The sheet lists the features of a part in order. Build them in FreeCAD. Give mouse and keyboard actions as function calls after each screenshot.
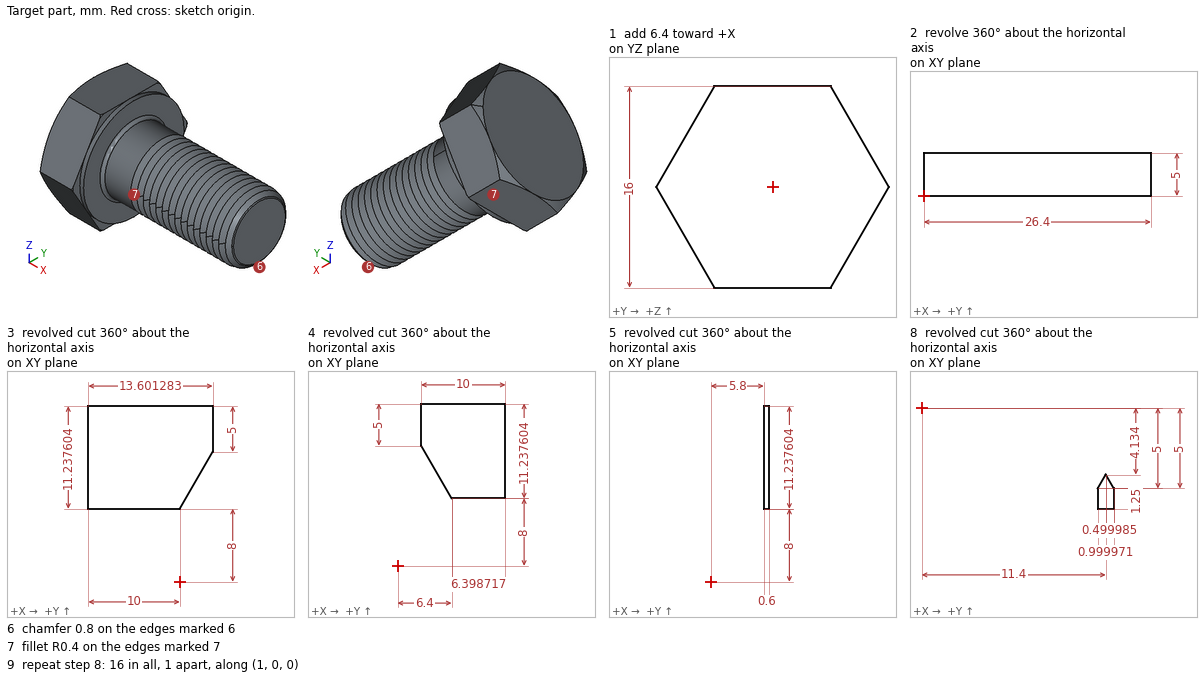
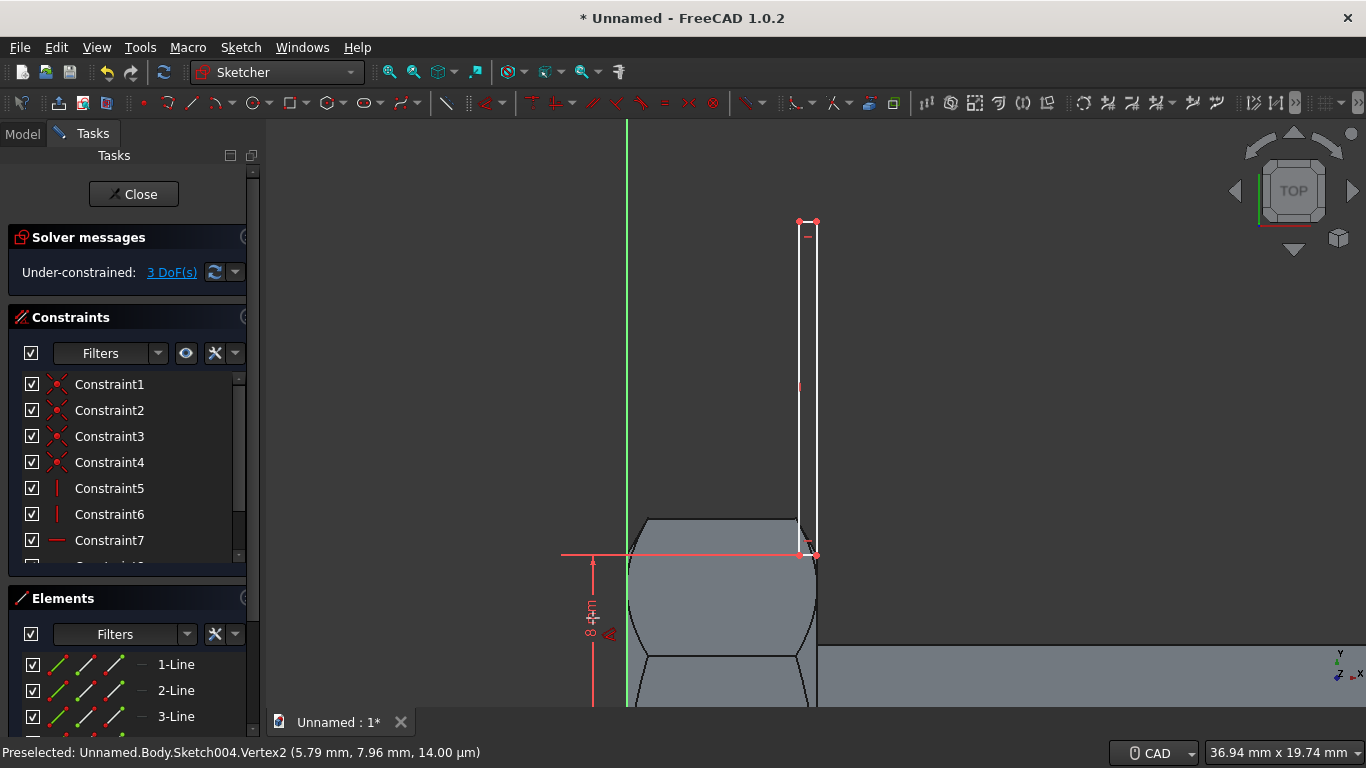
scroll(808, 555, up, 4)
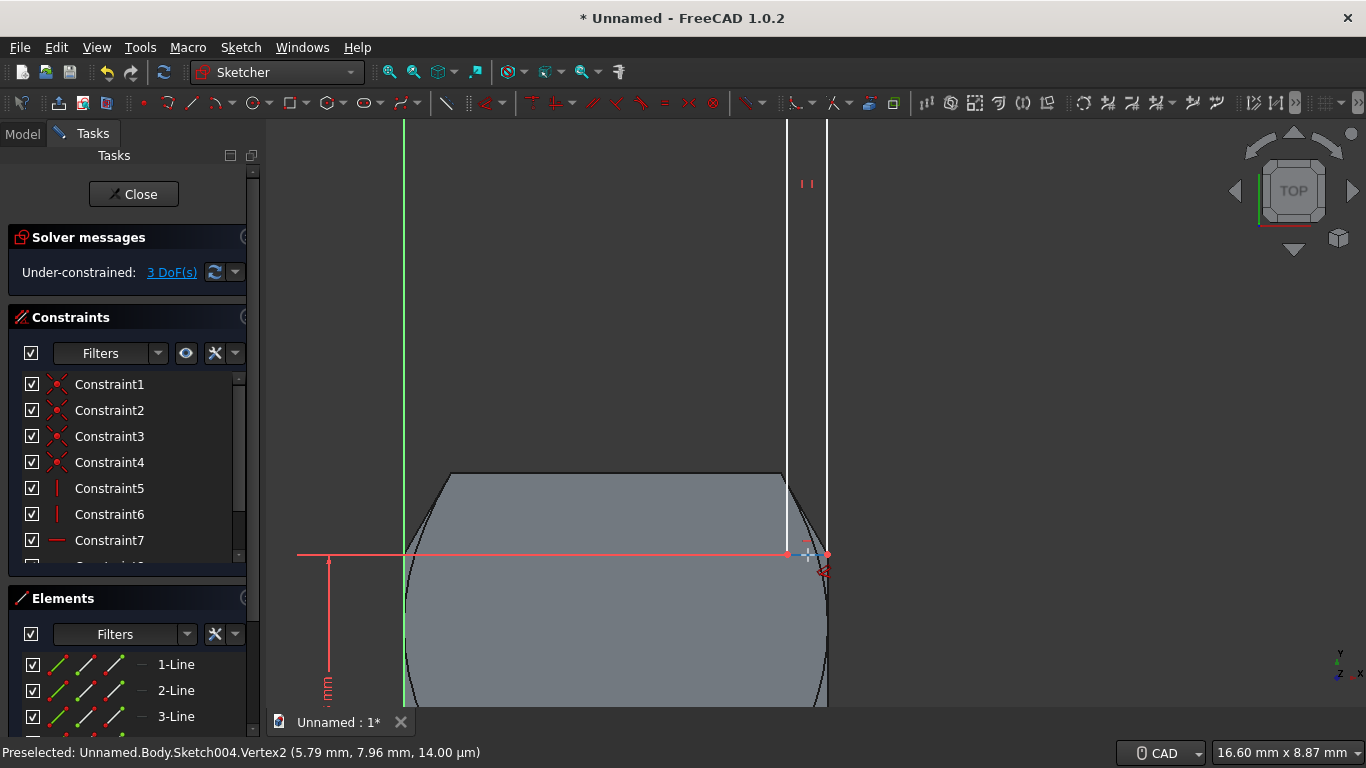
click(807, 555)
click(807, 589)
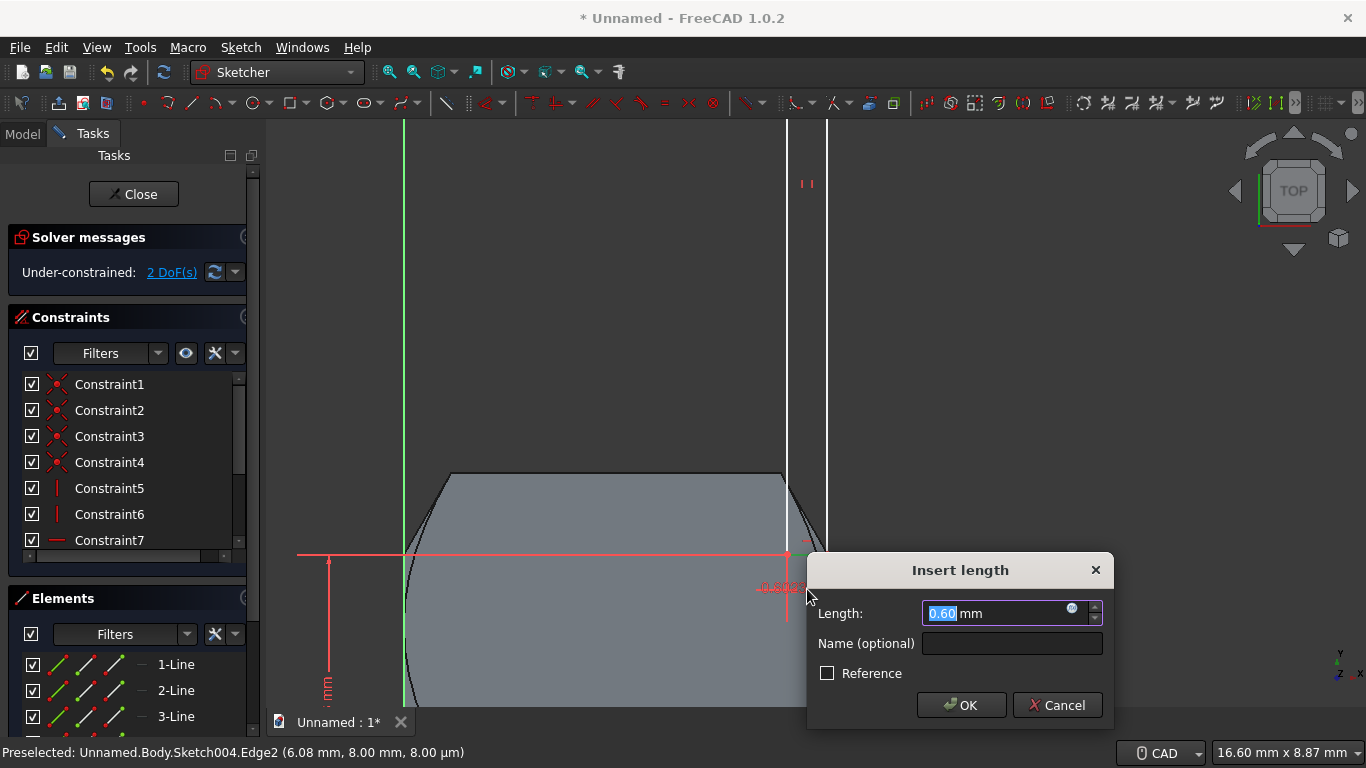
text(0.6)
key(Return)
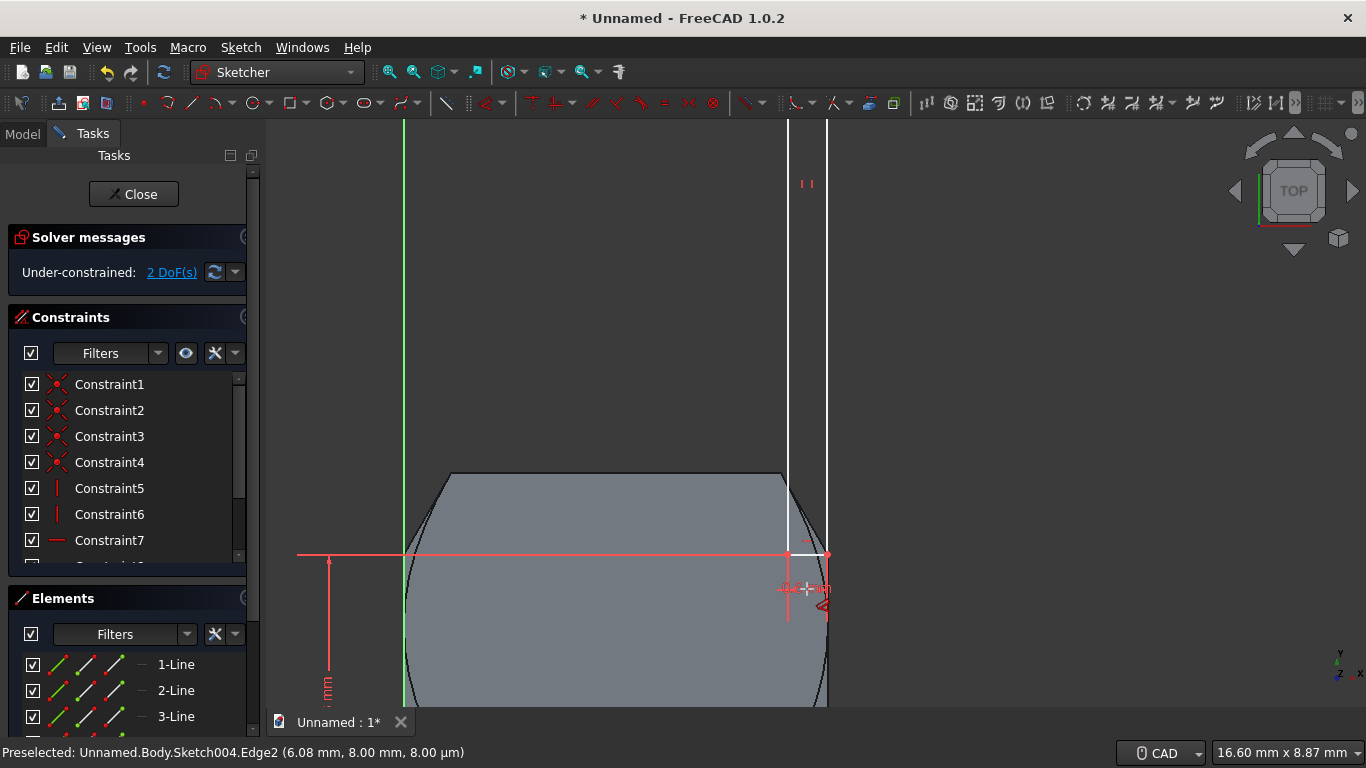
scroll(804, 398, down, 6)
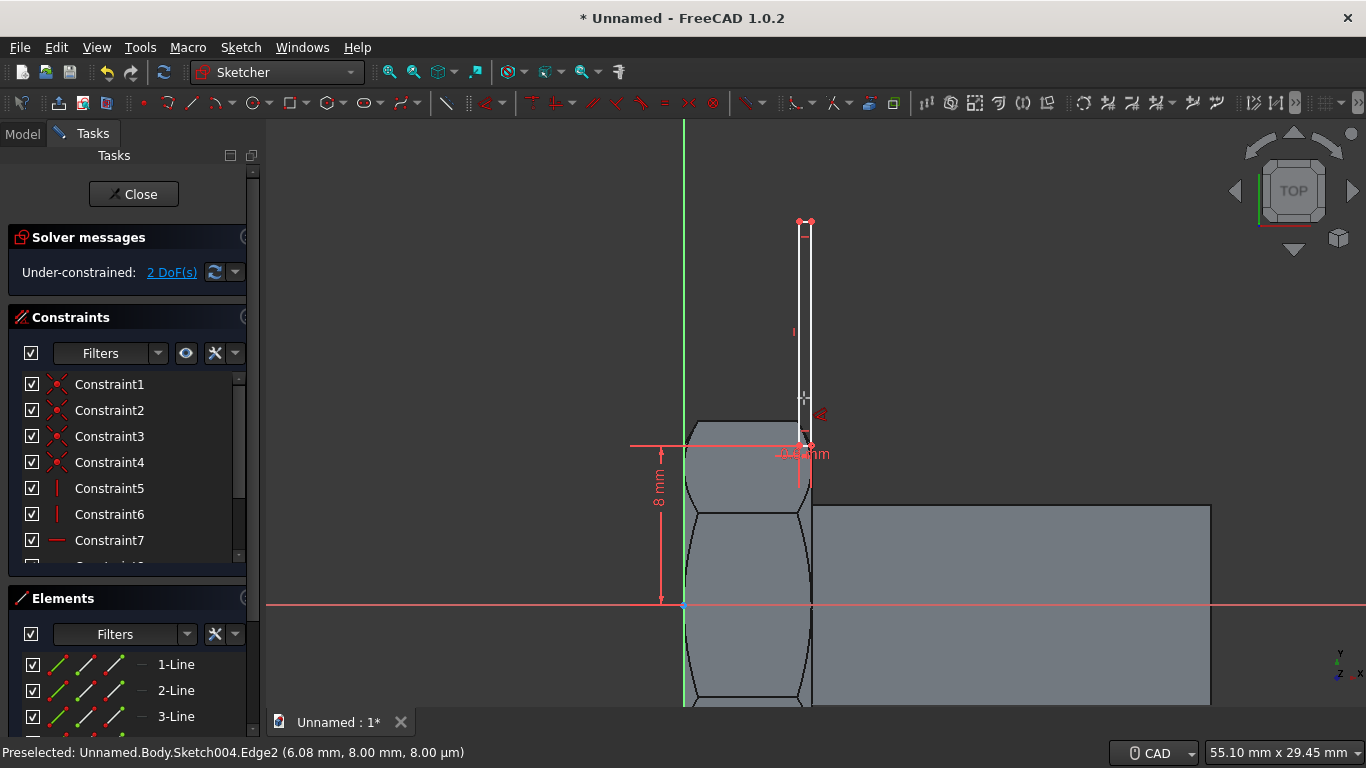
click(799, 222)
click(742, 639)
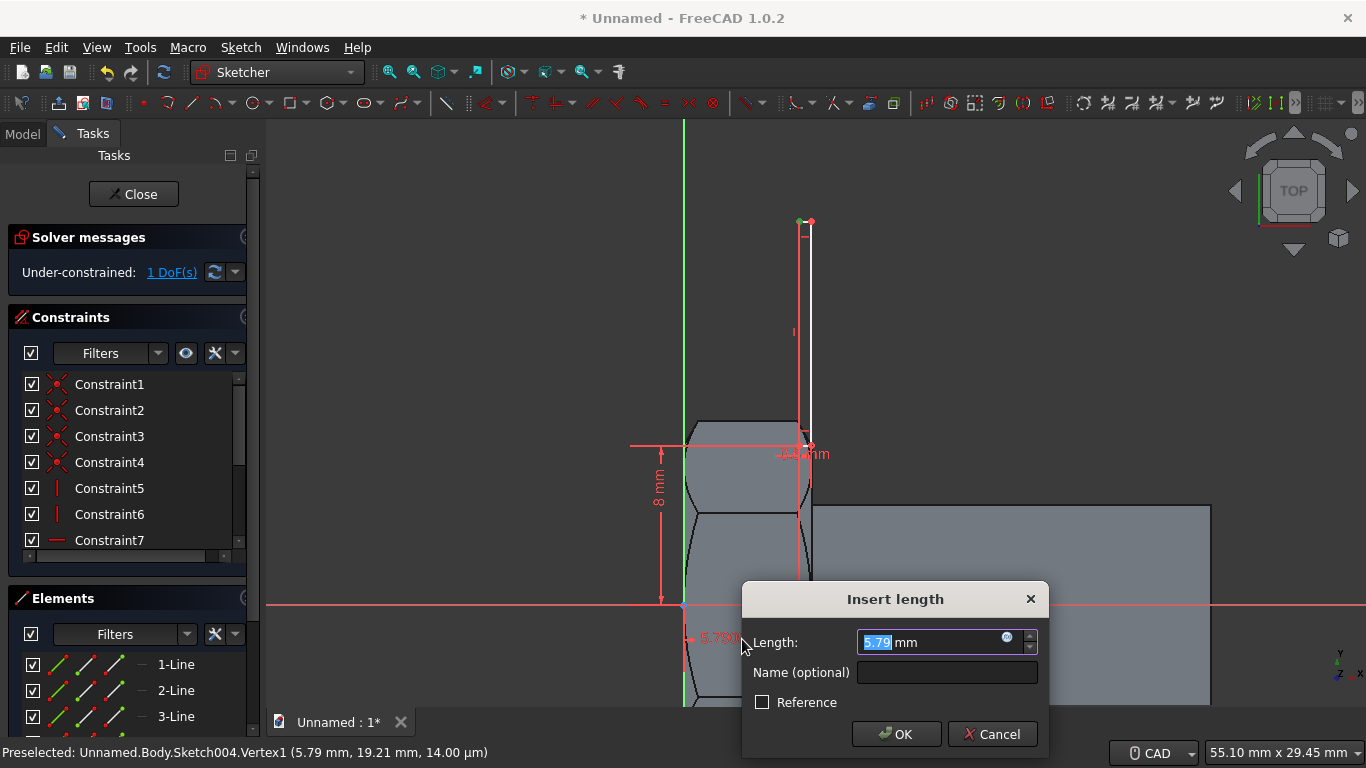
text(5.8)
key(Return)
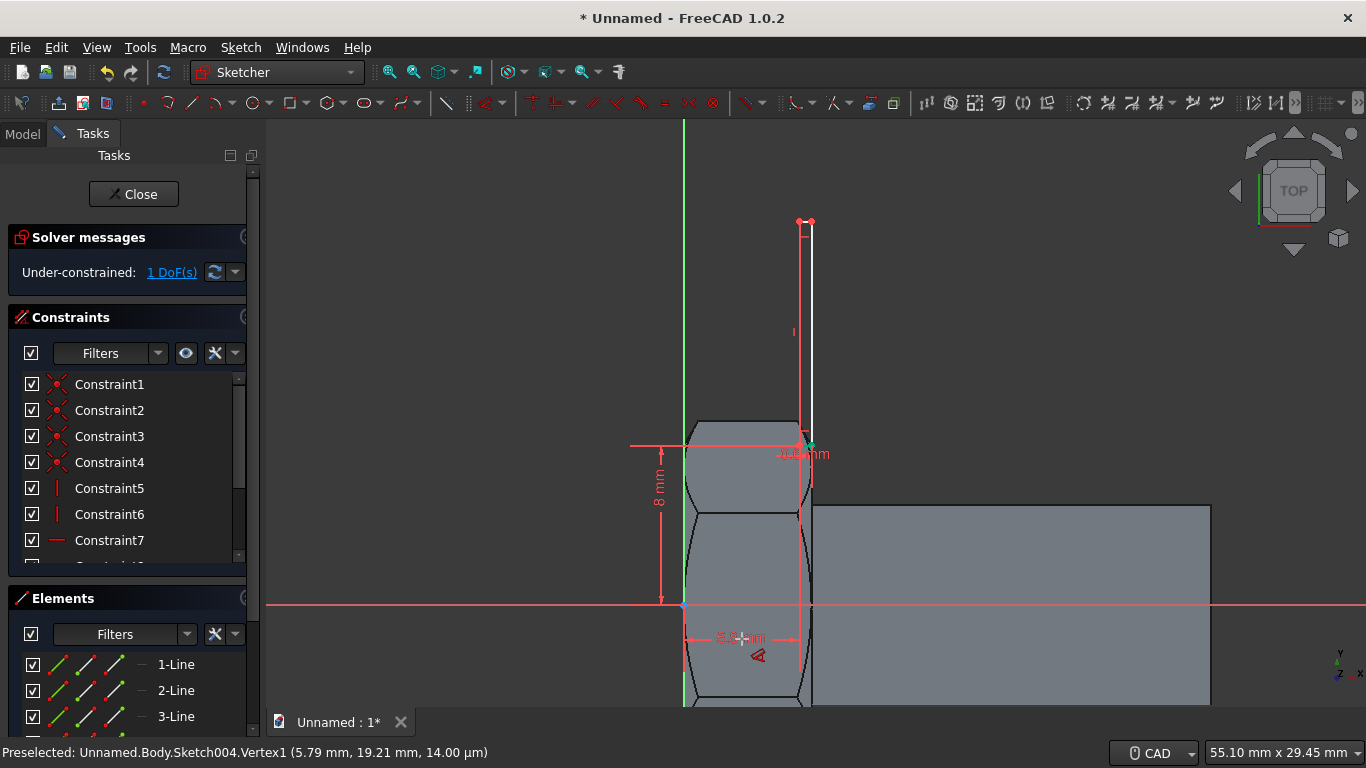
click(800, 289)
click(834, 334)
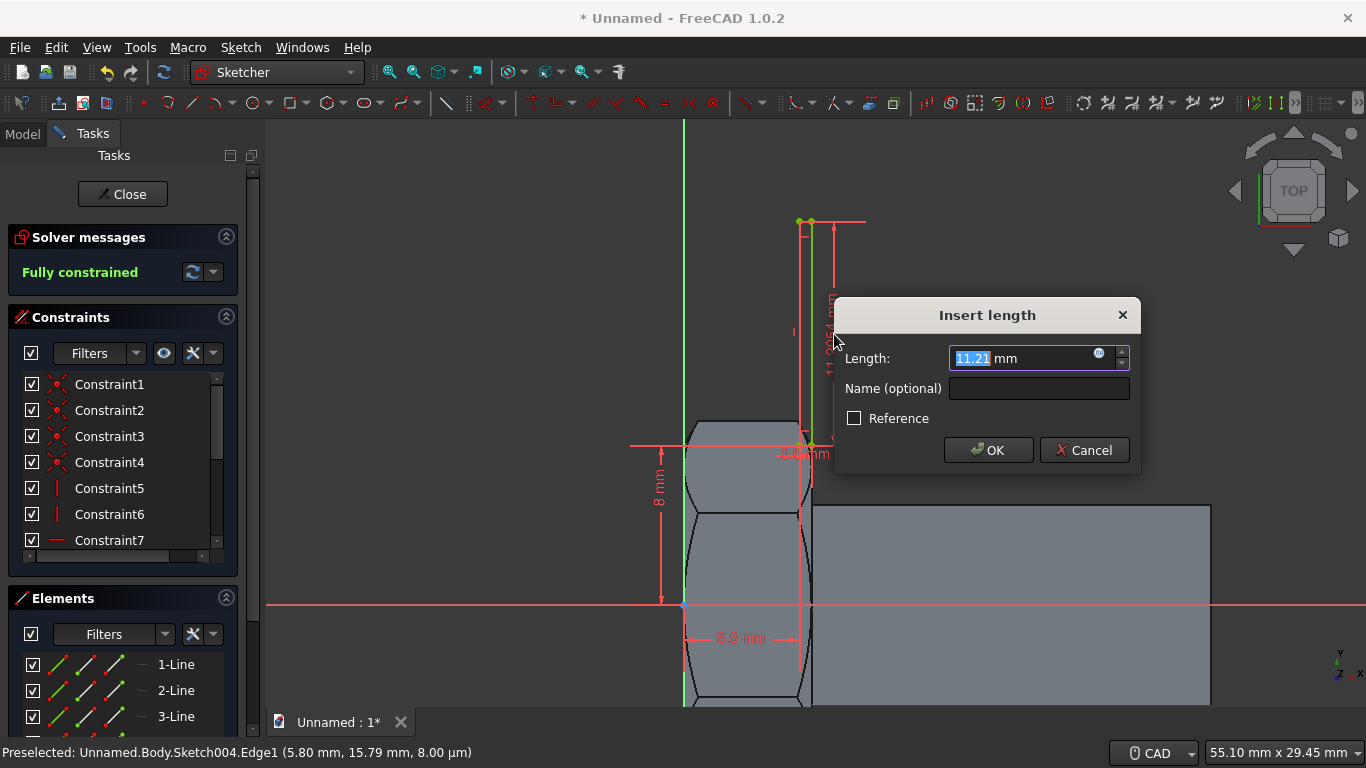
text(11.237604)
key(Return)
key(Escape)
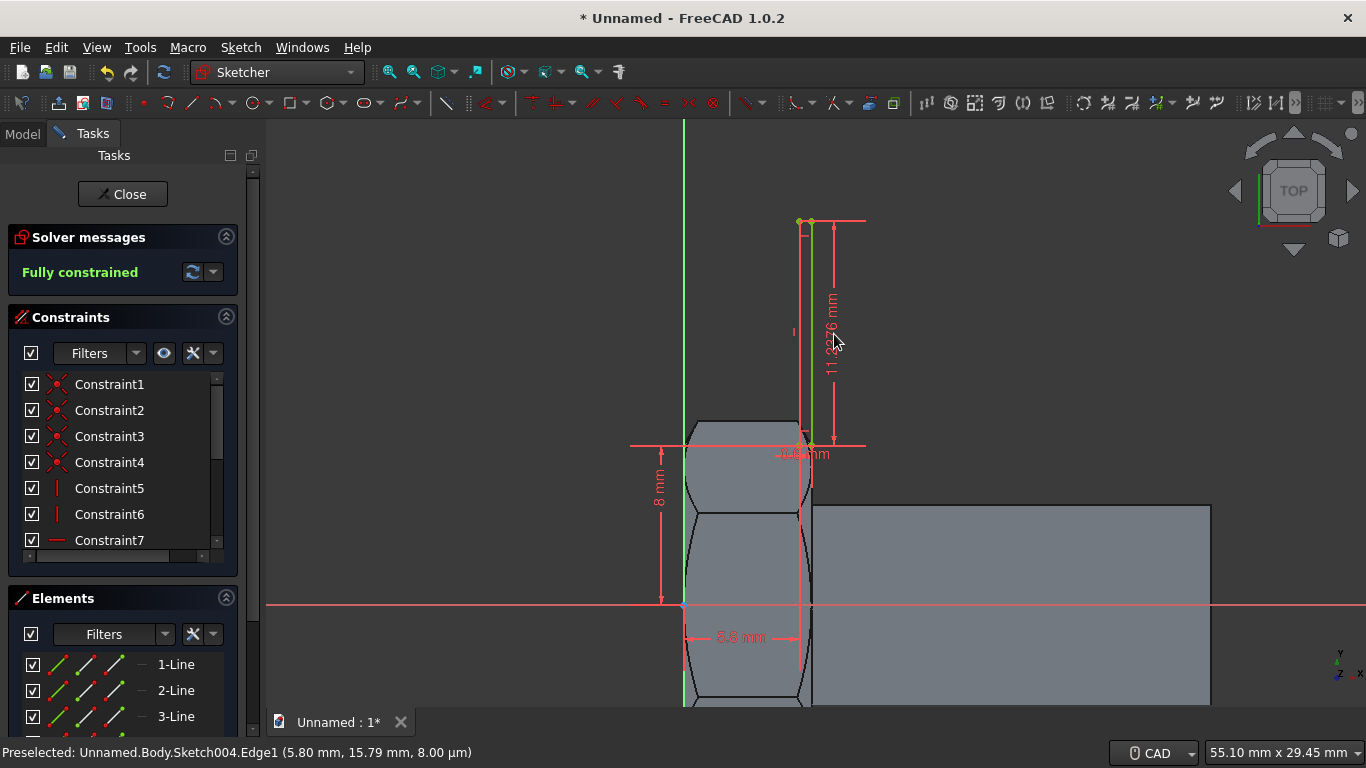
click(123, 194)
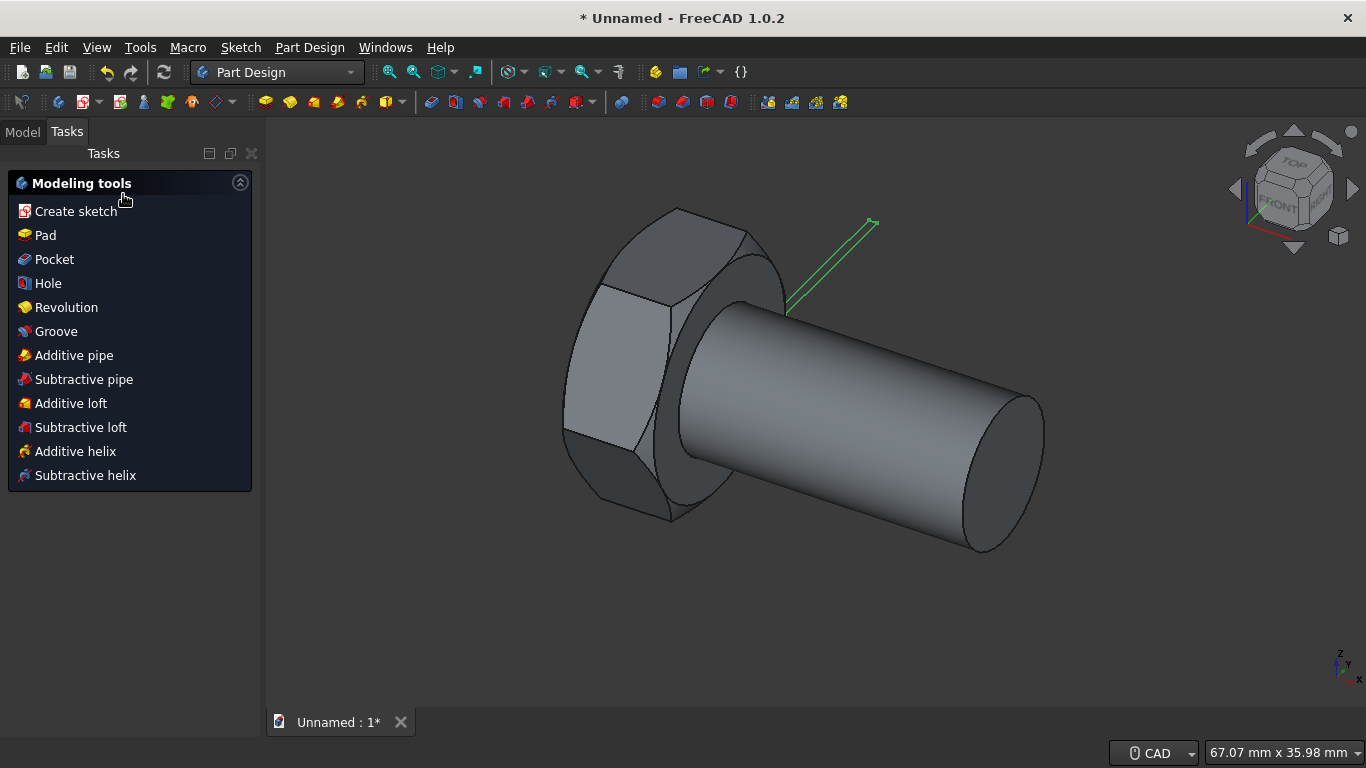
click(480, 102)